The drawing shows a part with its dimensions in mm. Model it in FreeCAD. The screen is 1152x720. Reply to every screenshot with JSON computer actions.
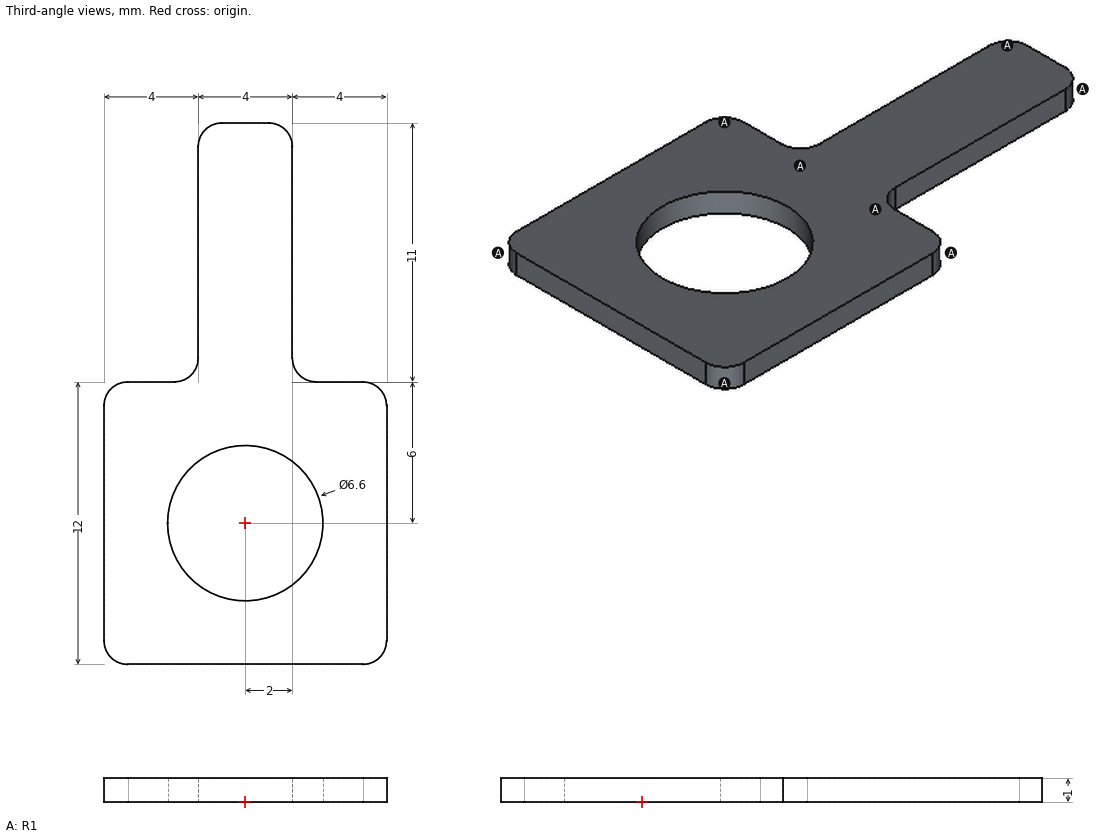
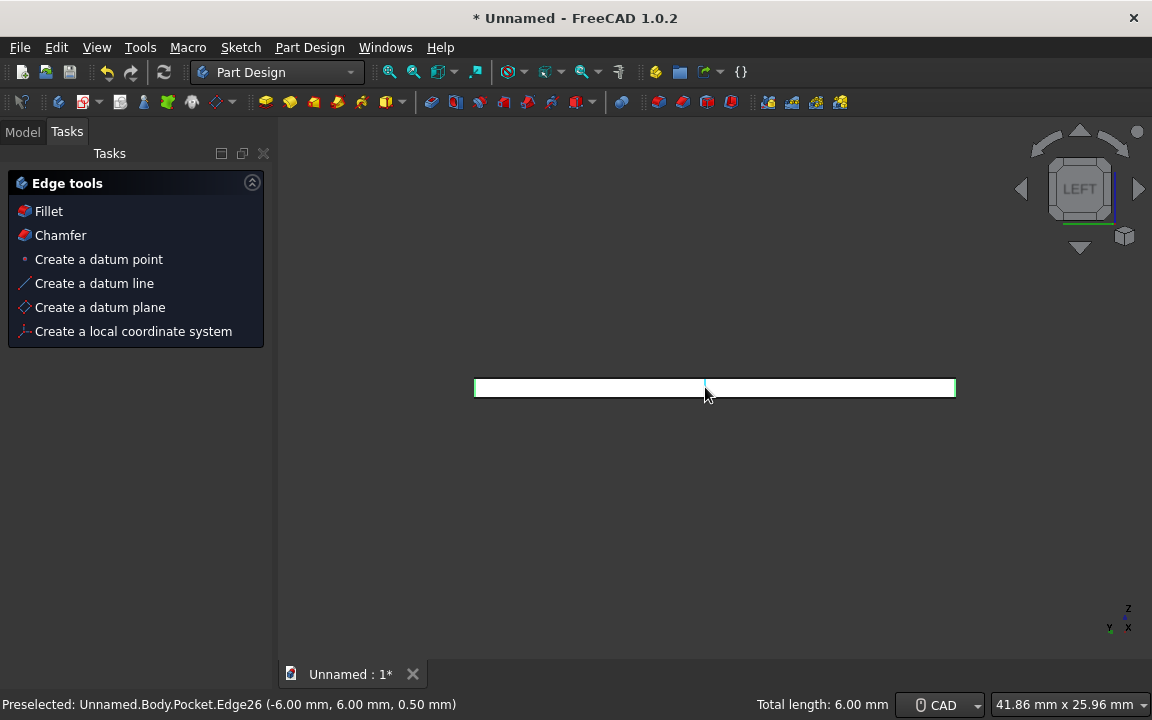
{"action": "key", "text": "v 3"}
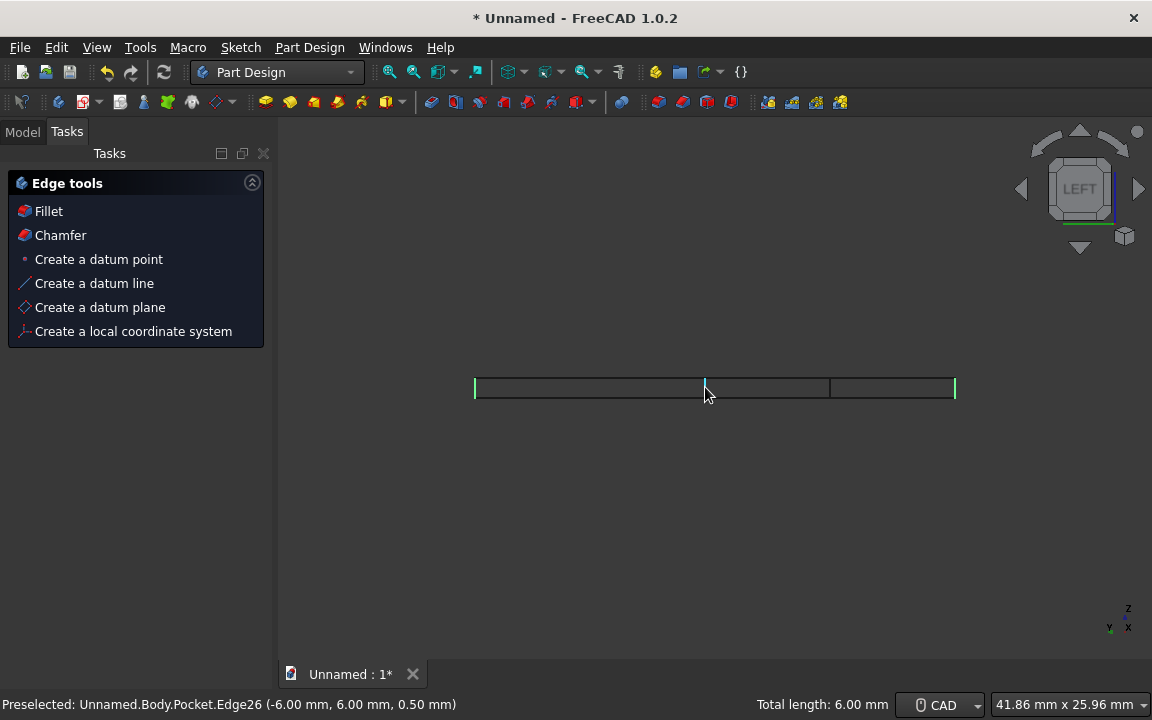
{"action": "key", "text": "0"}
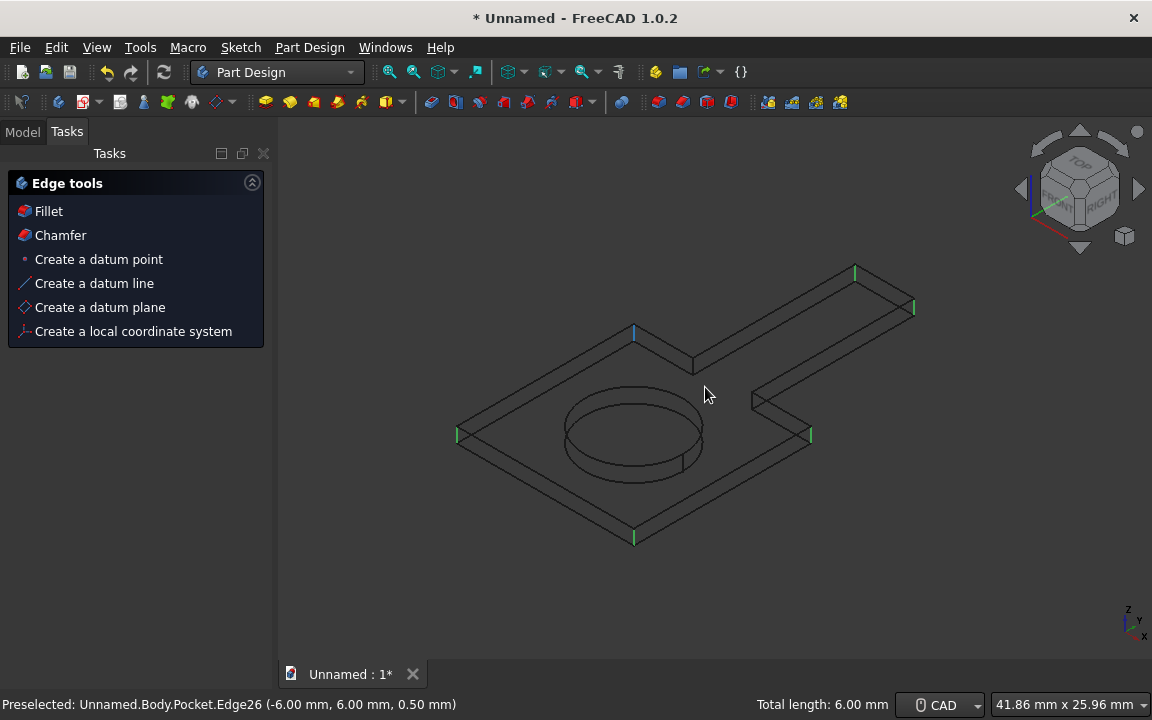
{"action": "left_click", "coordinate": [693, 366], "text": "ctrl"}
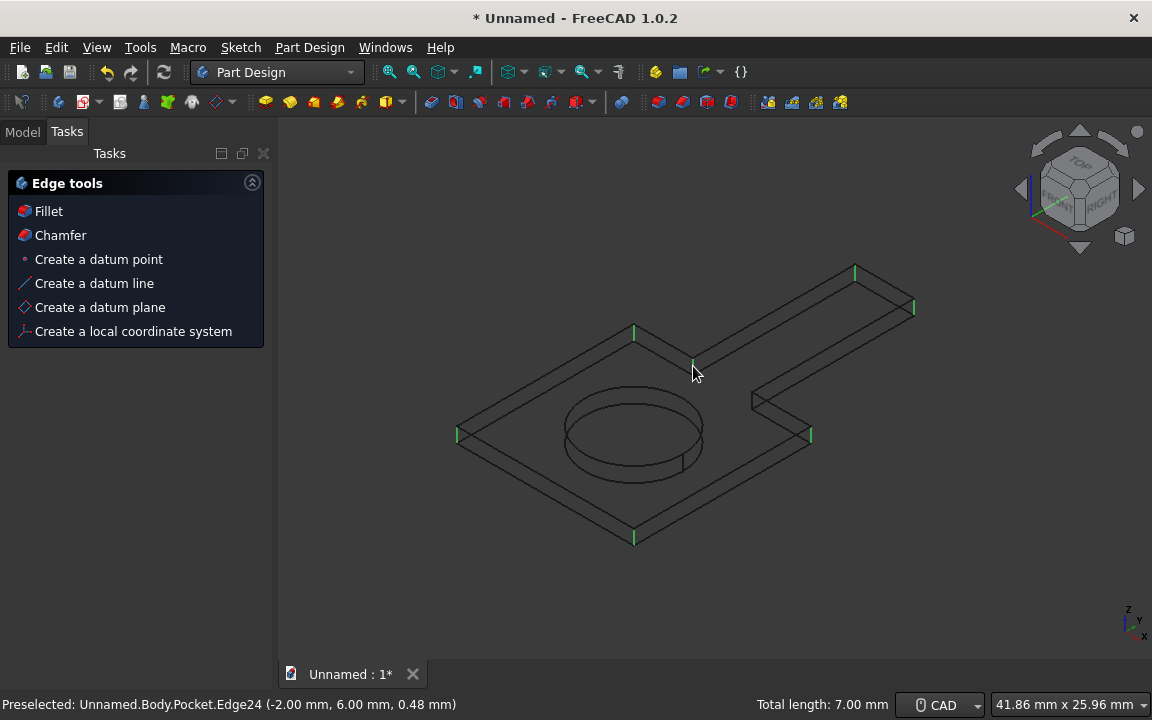
{"action": "left_click", "coordinate": [752, 400], "text": "ctrl"}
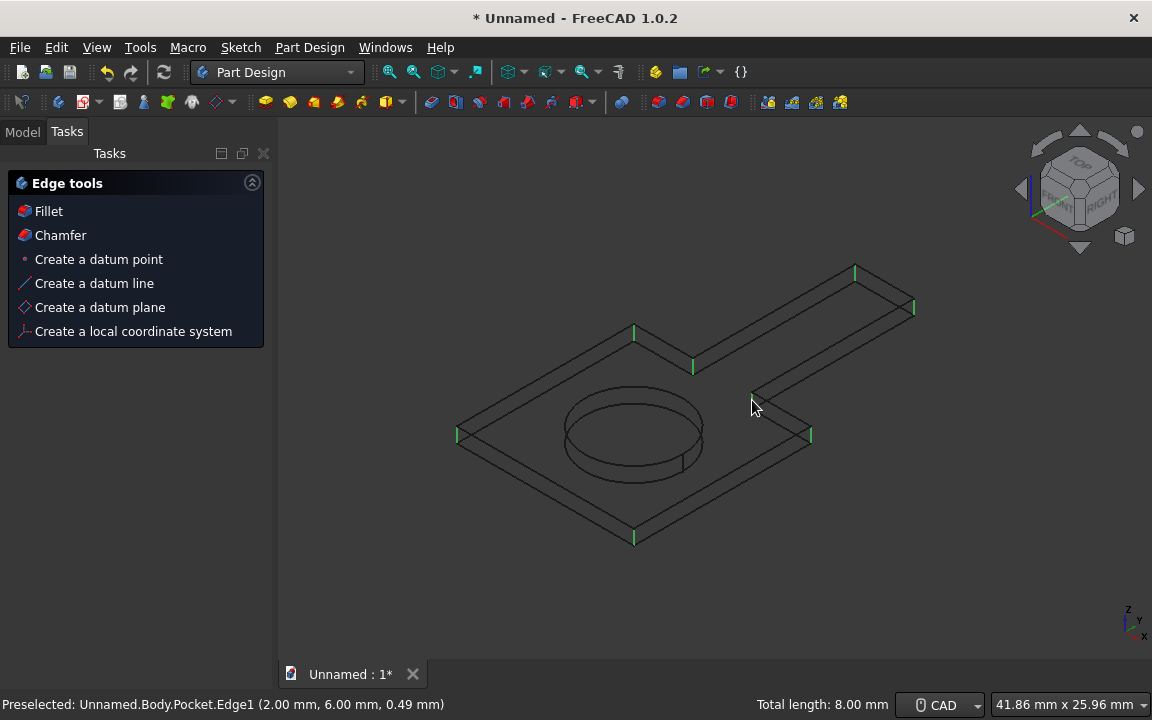
{"action": "key", "text": "v 1"}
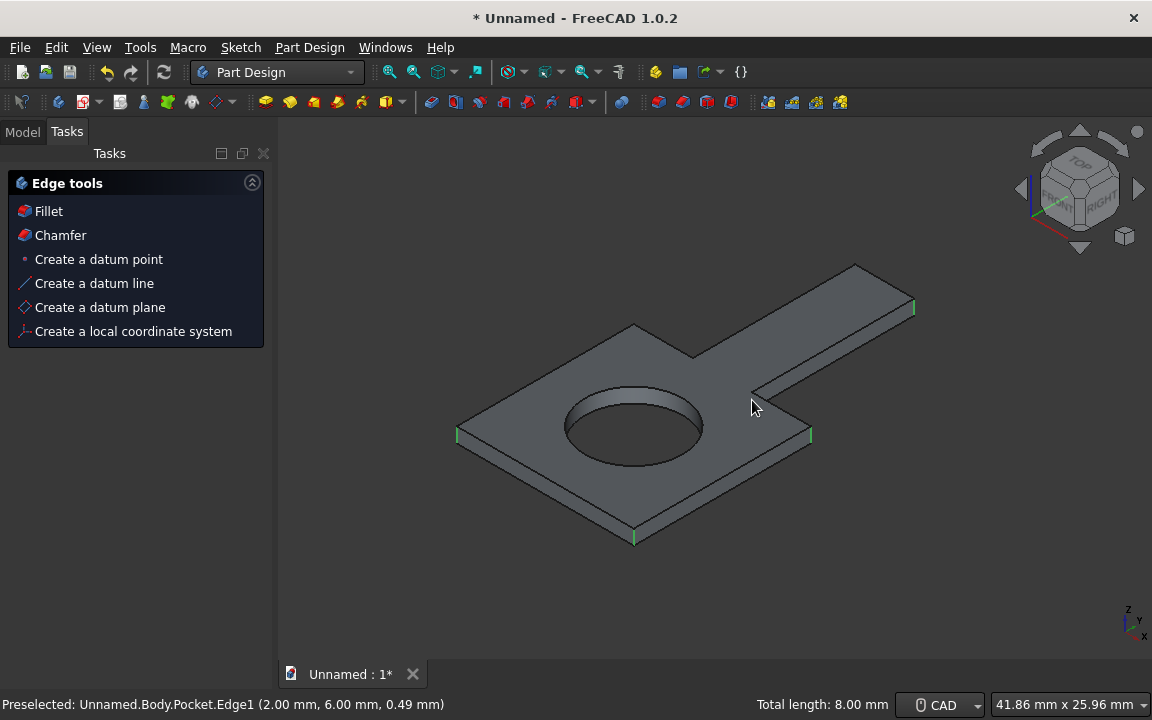
{"action": "left_click", "coordinate": [660, 102]}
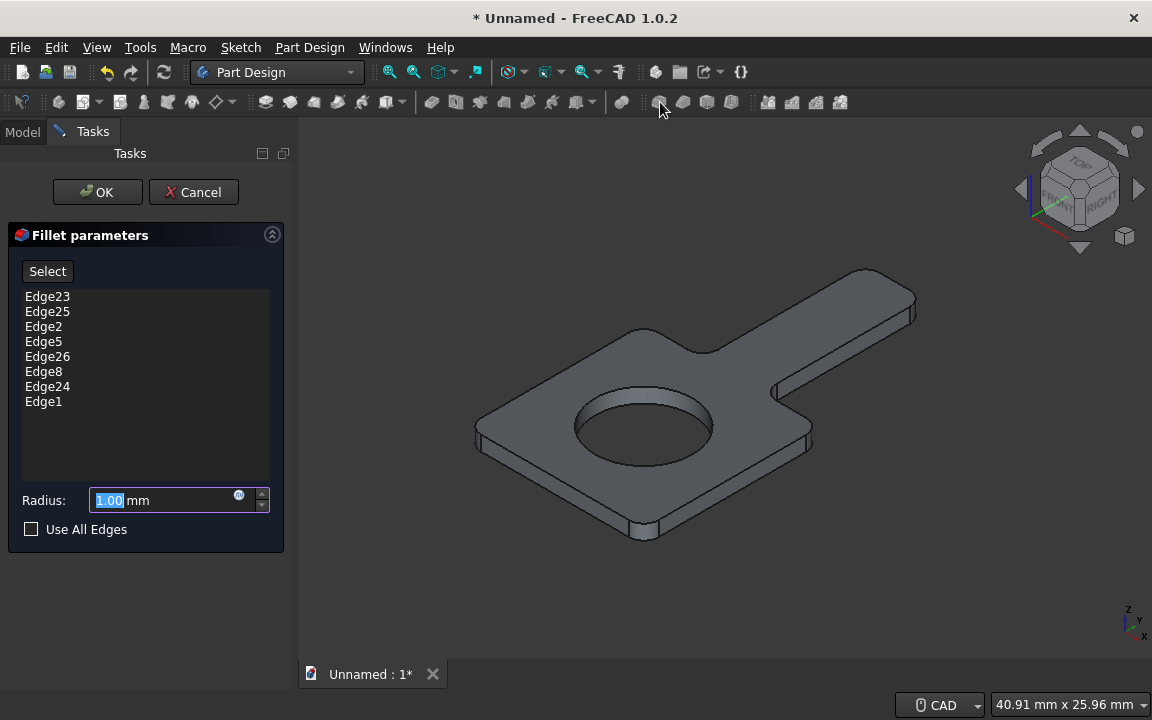
{"action": "type", "text": "1"}
{"action": "key", "text": "Tab"}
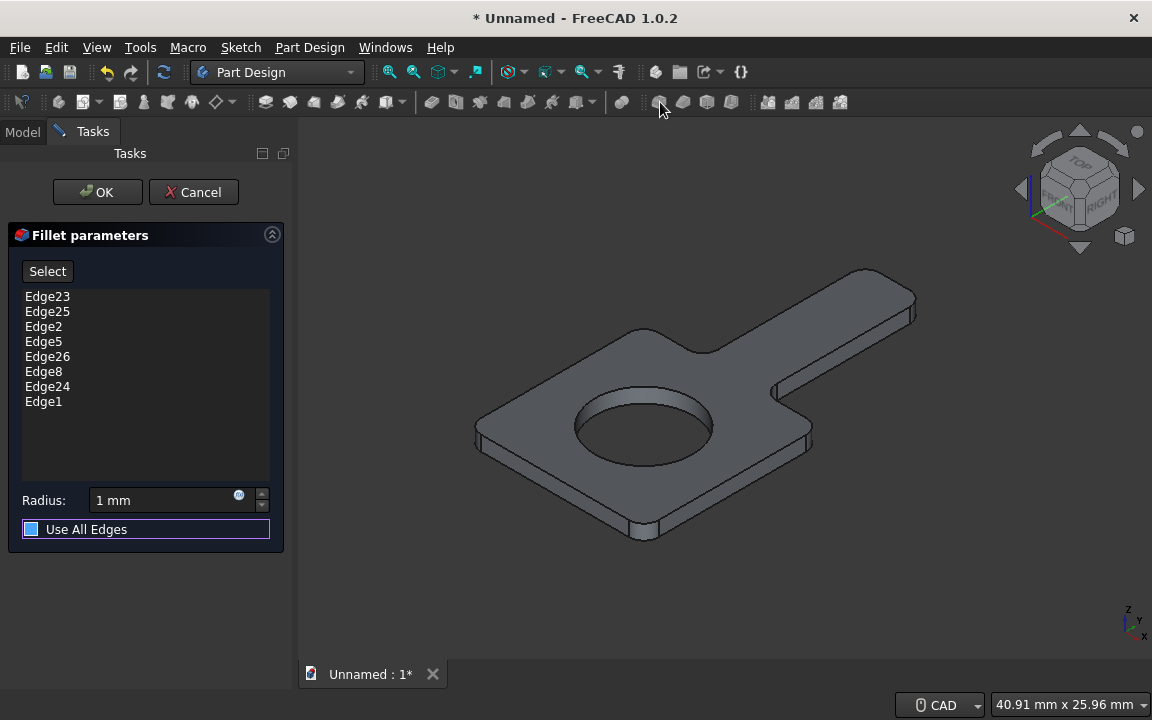
{"action": "left_click", "coordinate": [98, 192]}